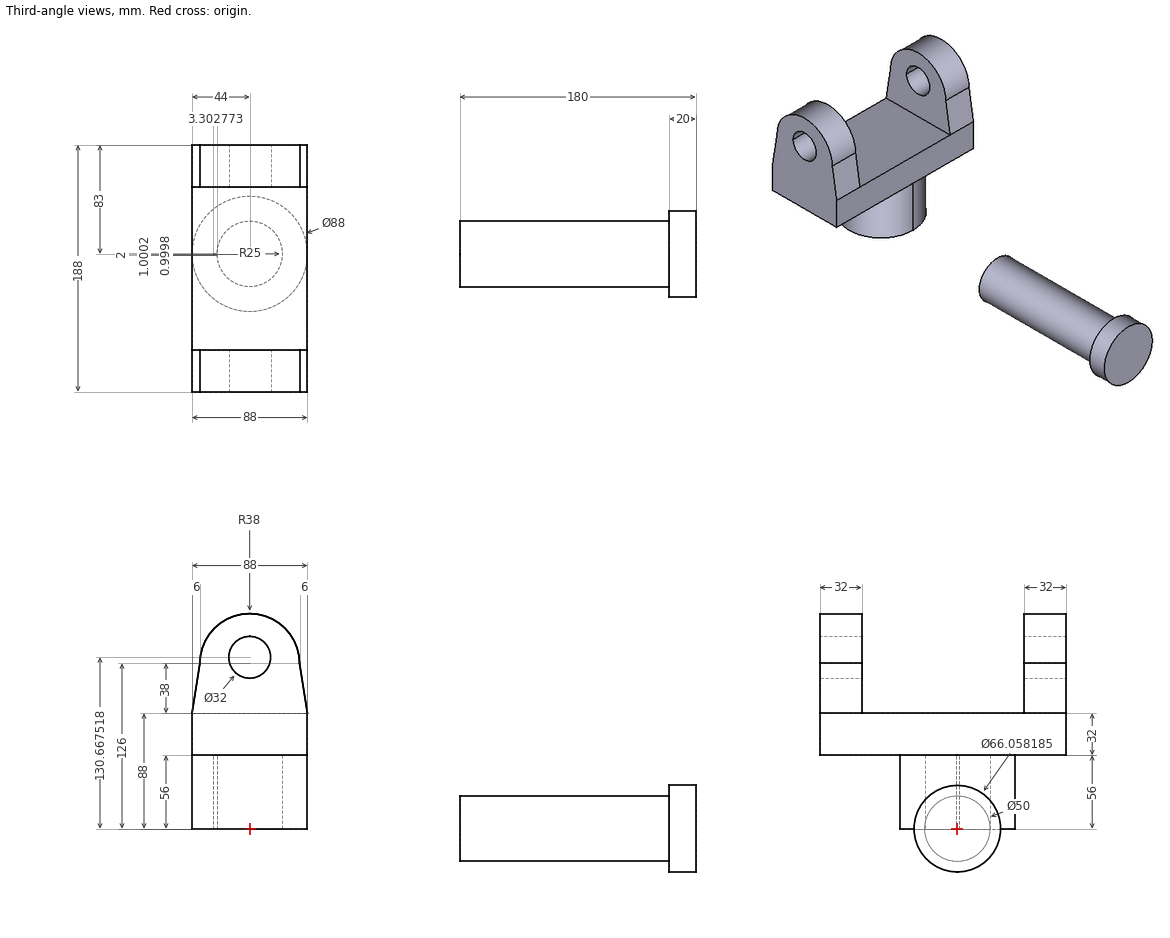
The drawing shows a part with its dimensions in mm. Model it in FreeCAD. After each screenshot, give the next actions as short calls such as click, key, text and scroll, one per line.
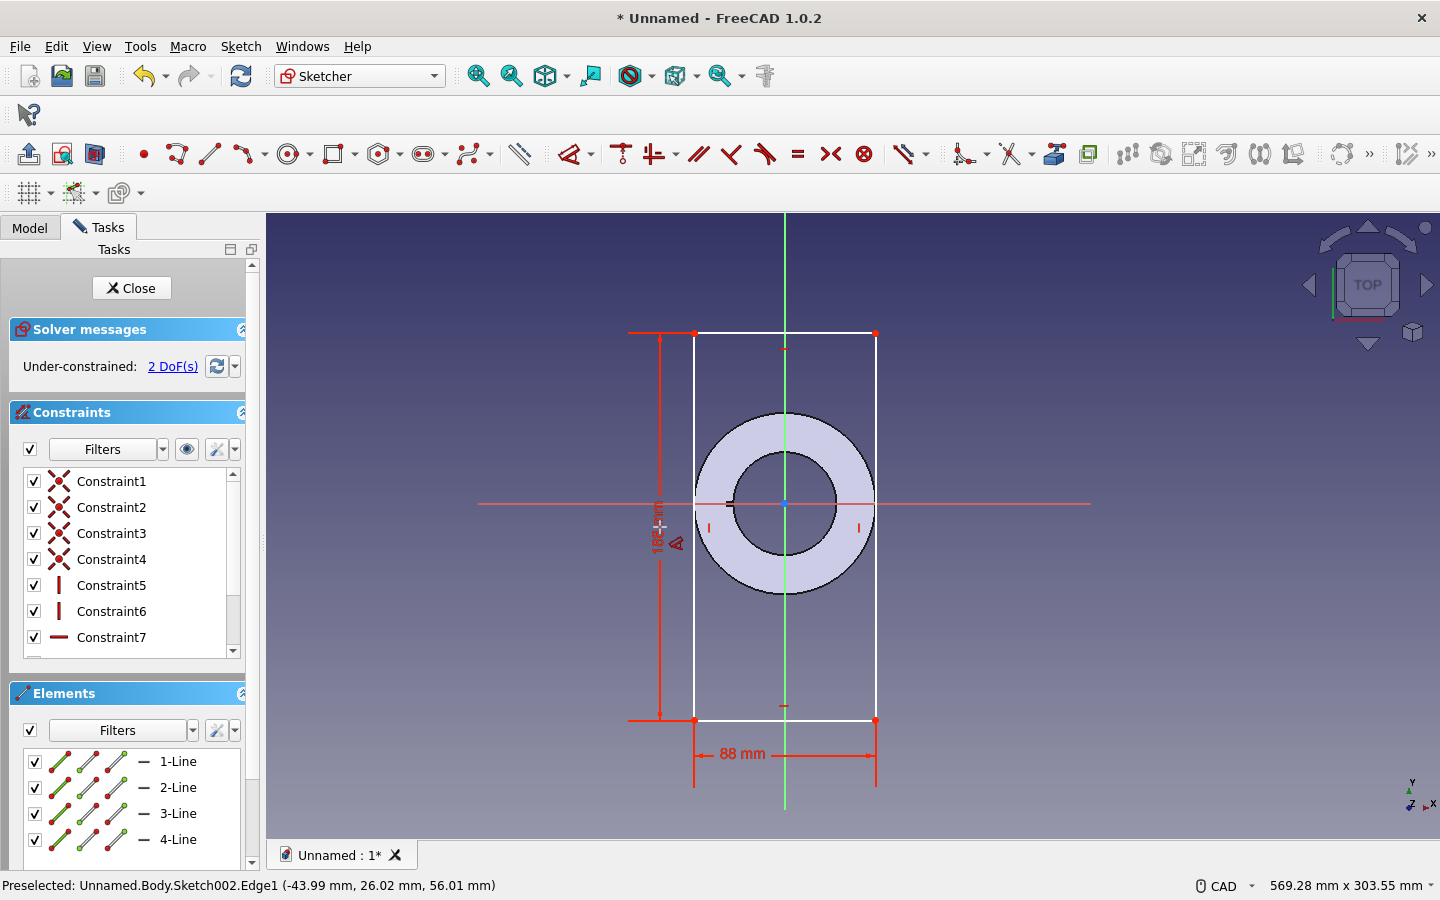
click(694, 333)
click(740, 299)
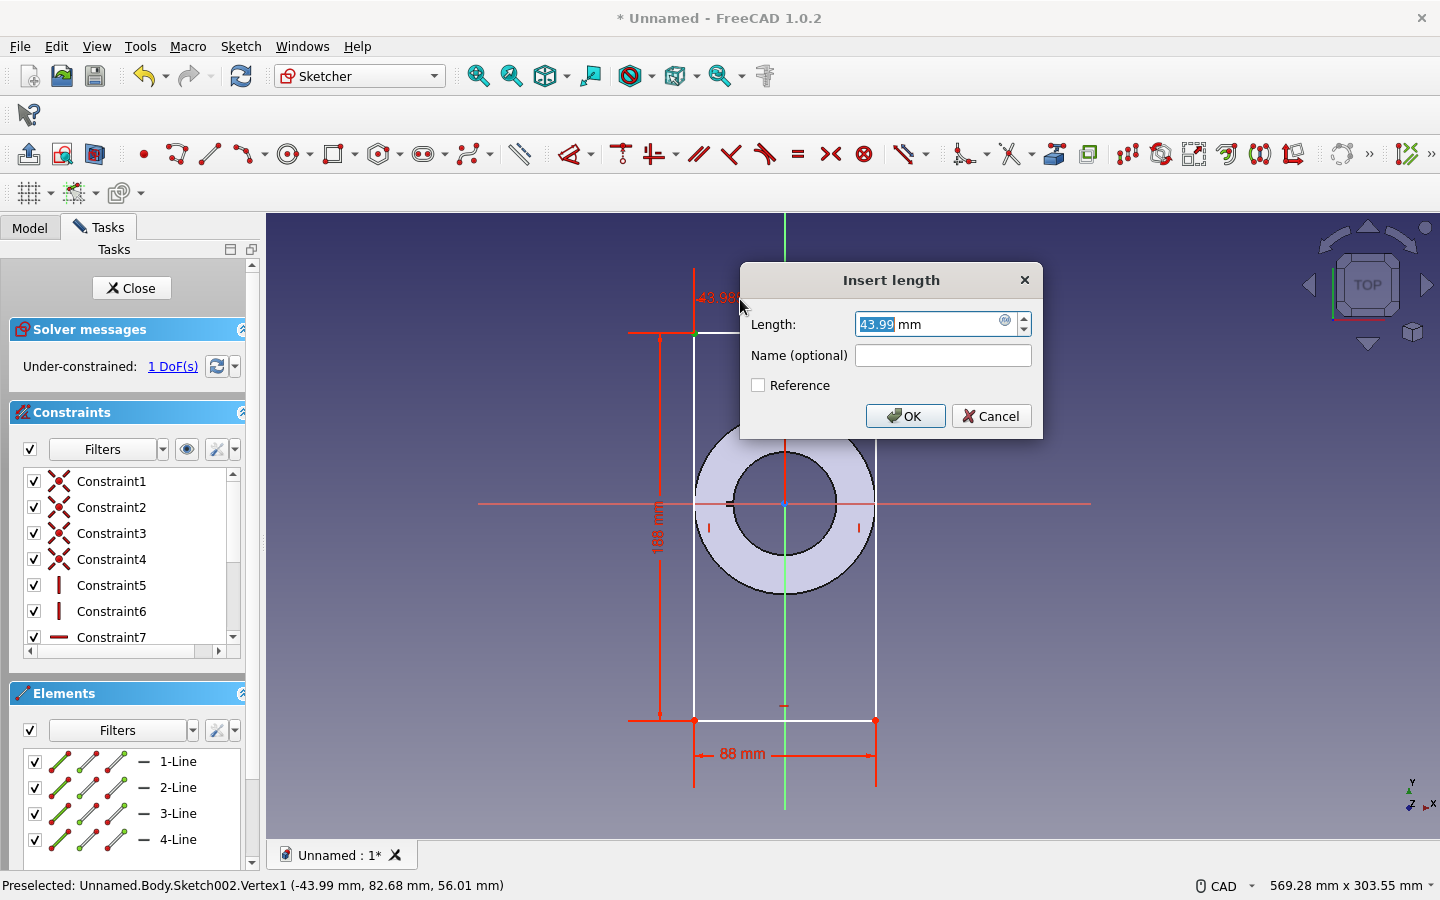
text(44)
key(Return)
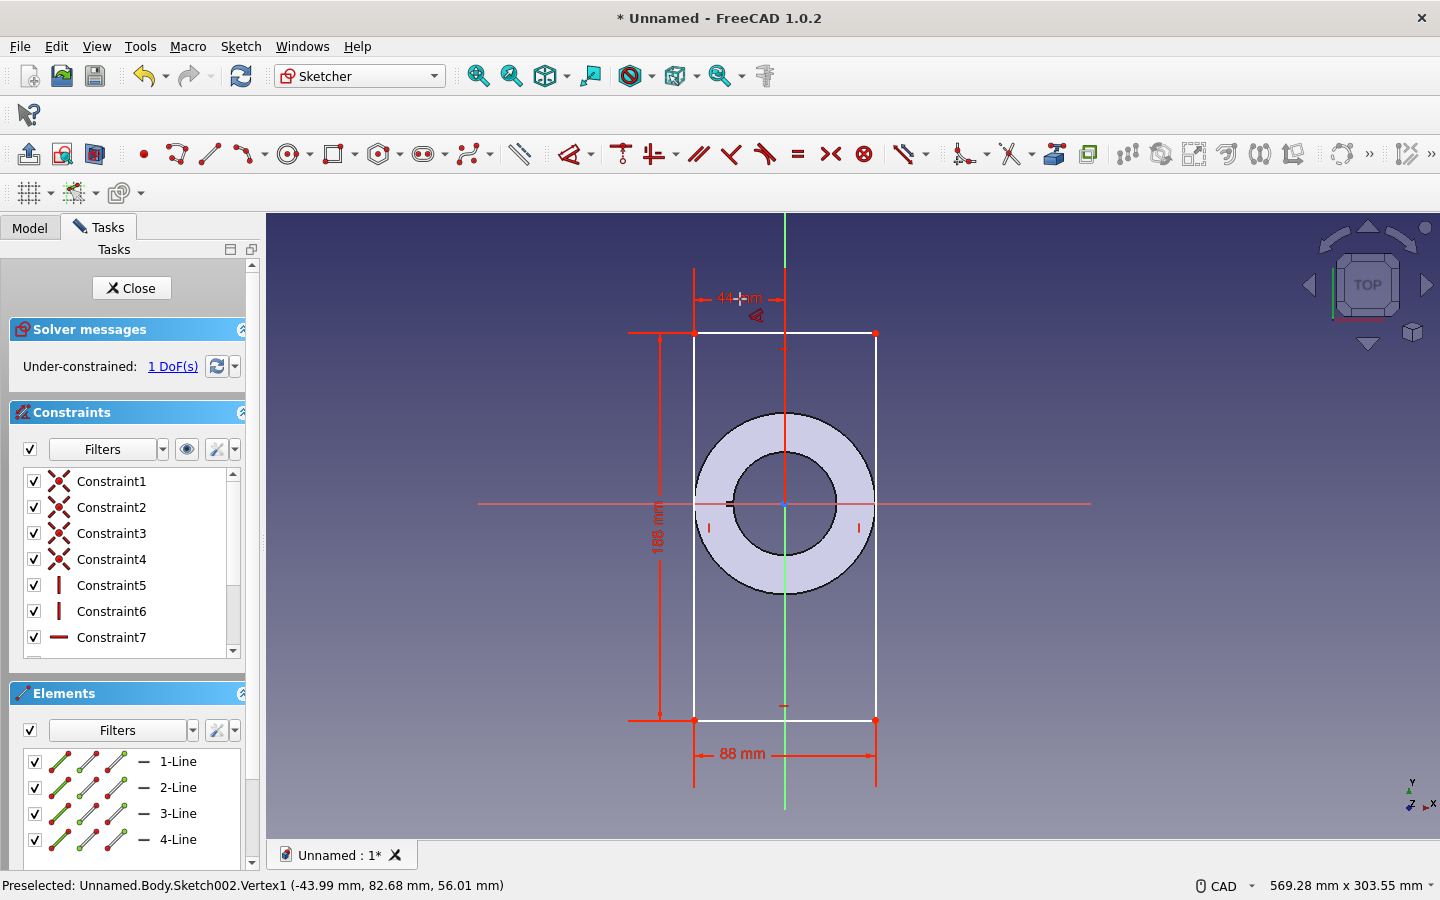
click(694, 333)
click(660, 418)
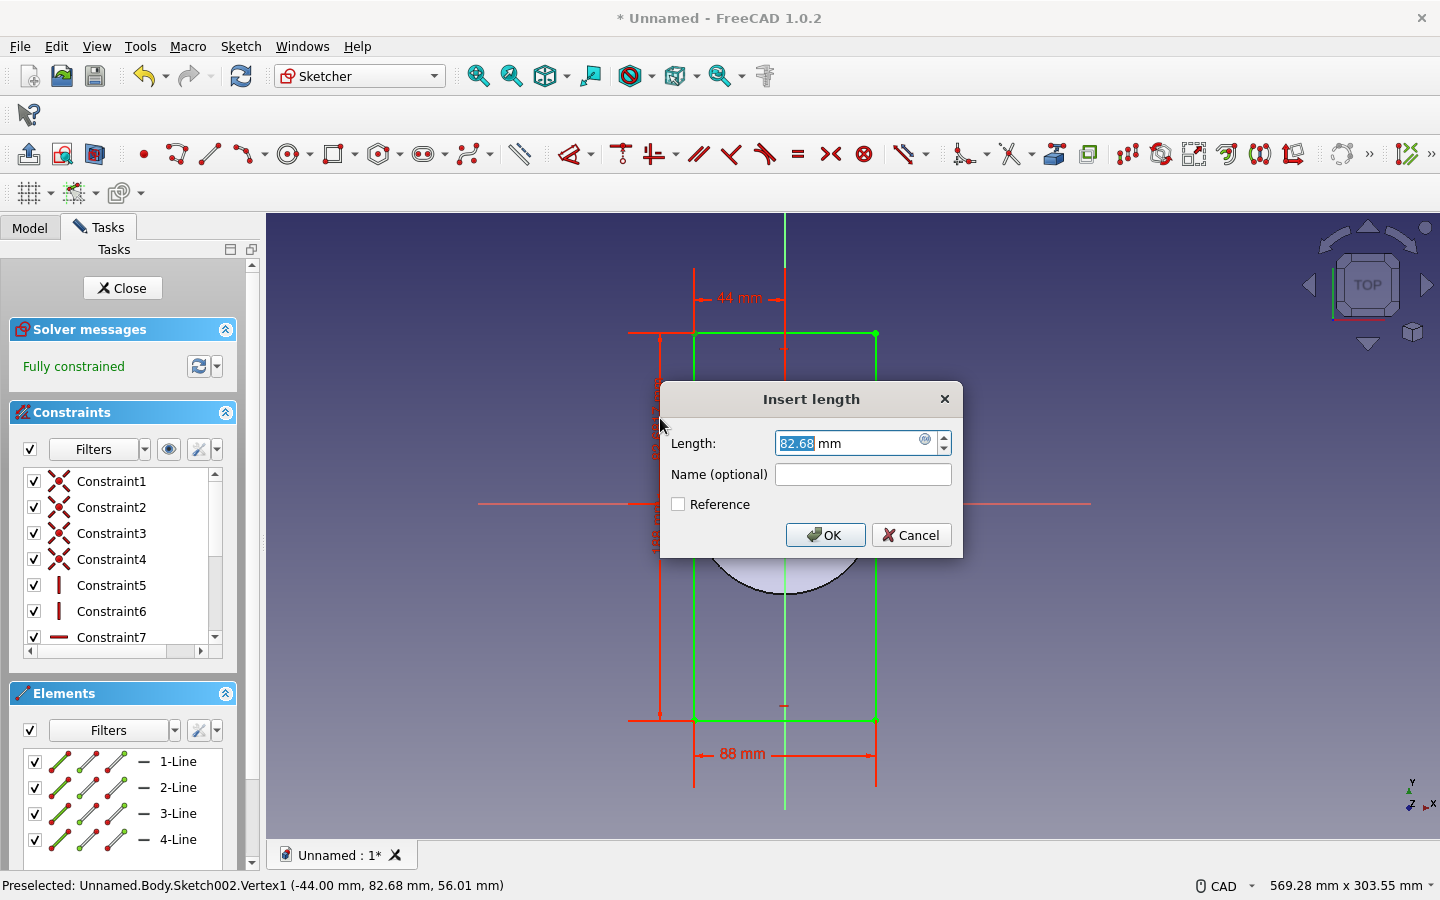
text(83)
key(Return)
key(Escape)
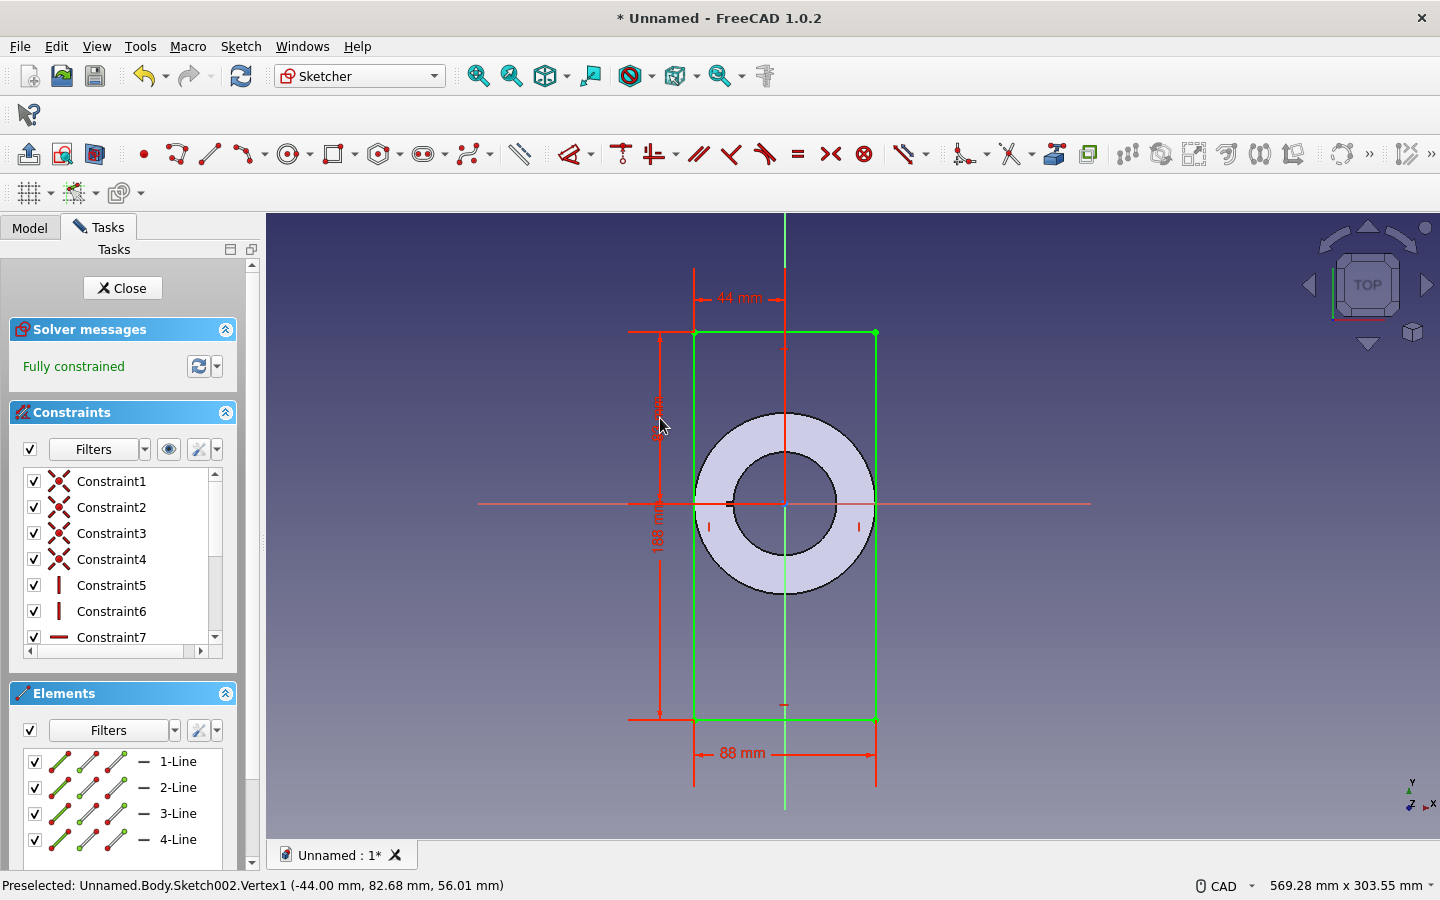
click(123, 288)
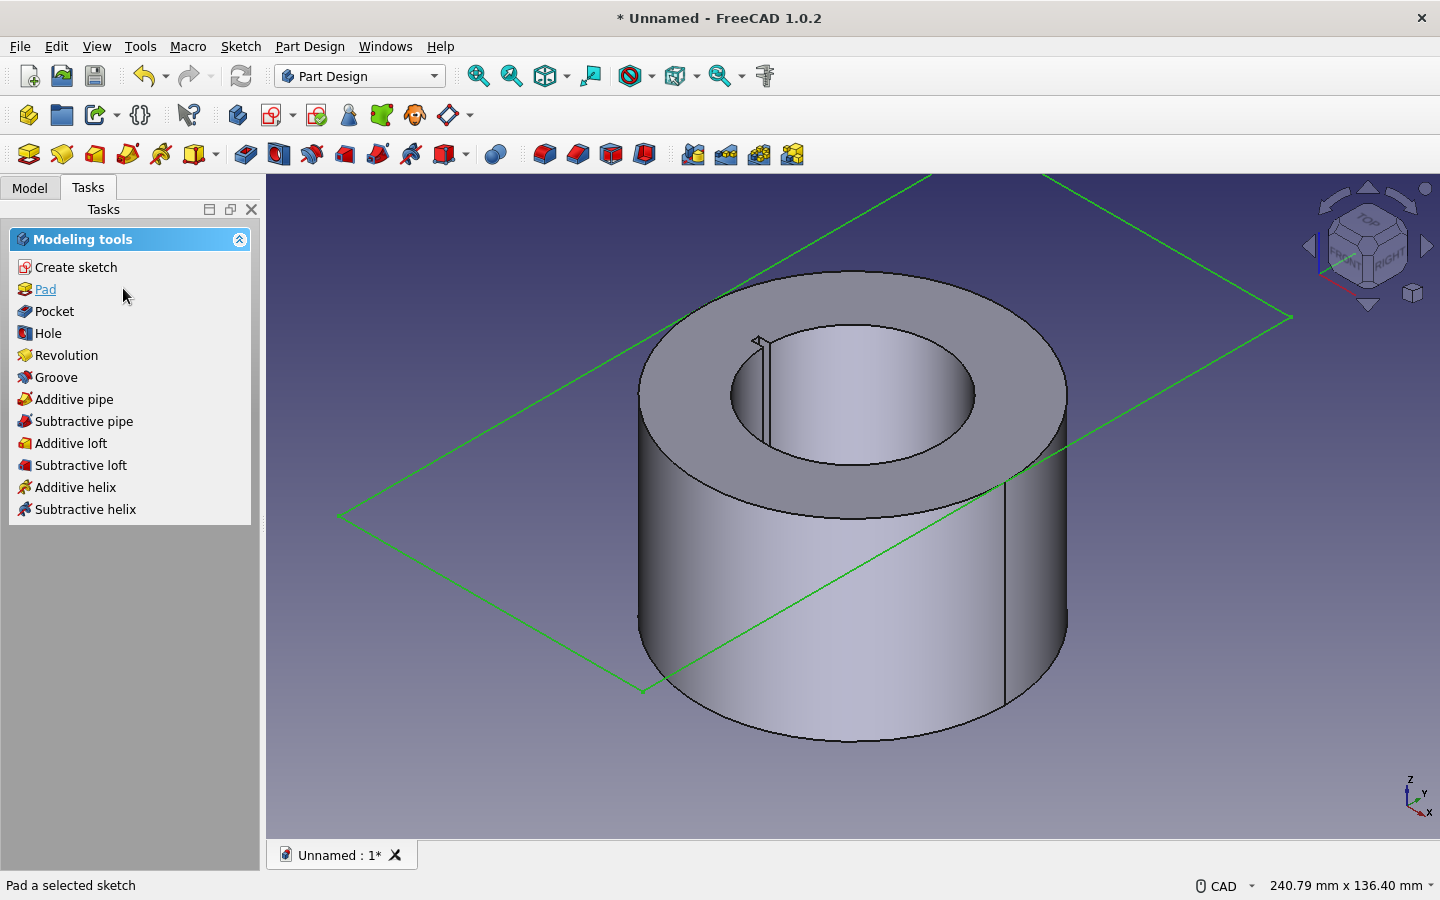
click(29, 154)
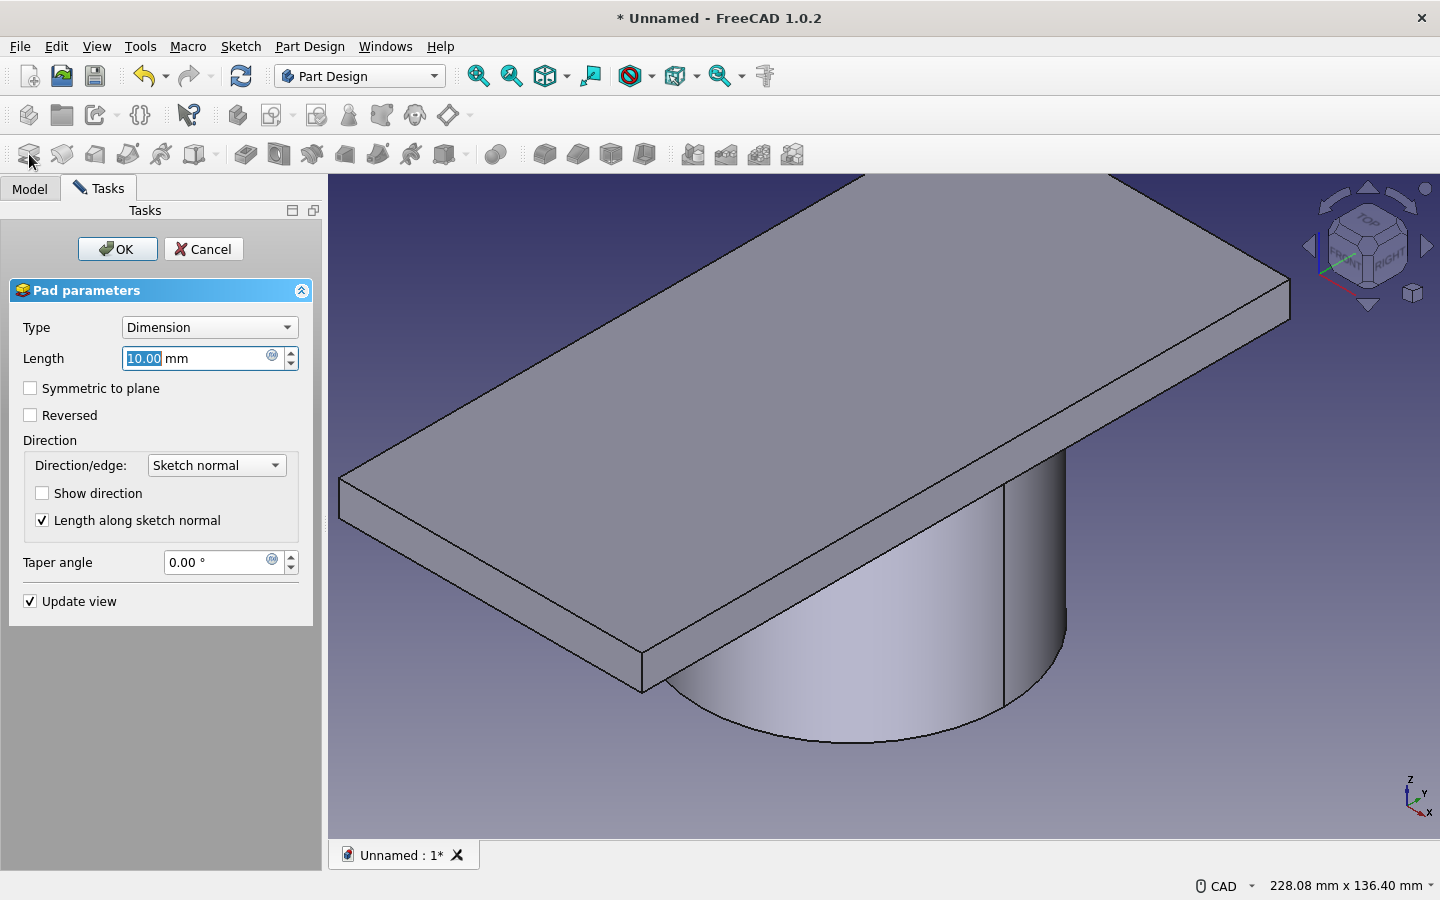
text(32)
key(Tab)